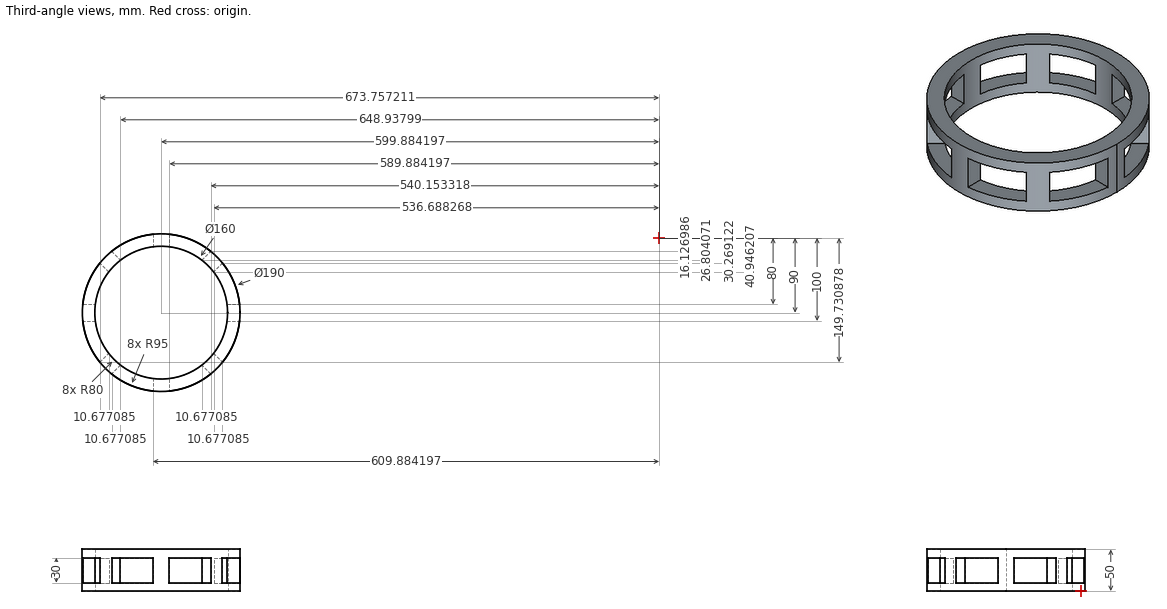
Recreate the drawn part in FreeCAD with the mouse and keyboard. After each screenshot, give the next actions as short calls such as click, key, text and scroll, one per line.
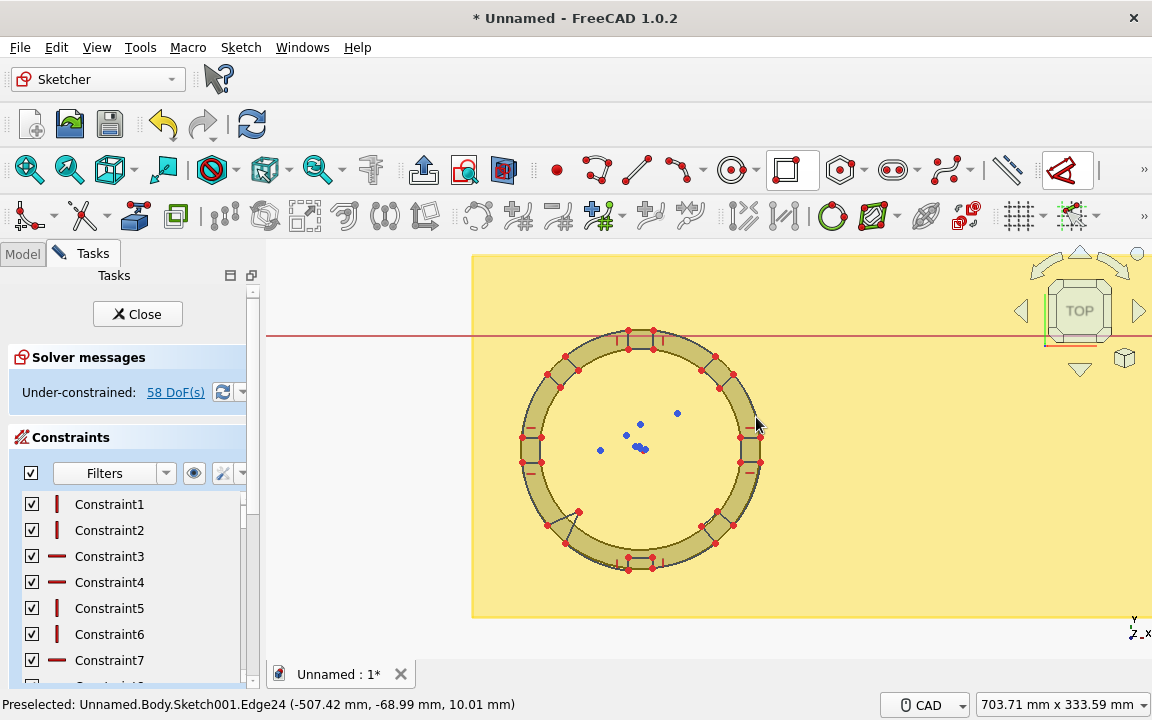
scroll(579, 512, up, 15)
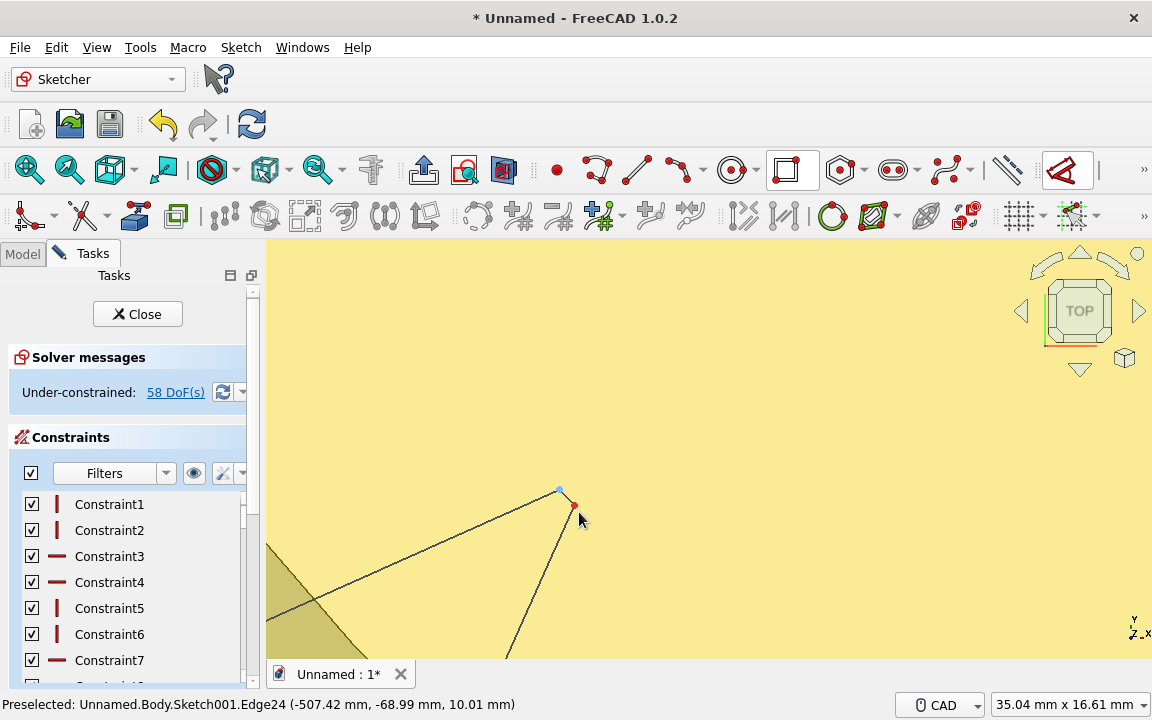
click(567, 497)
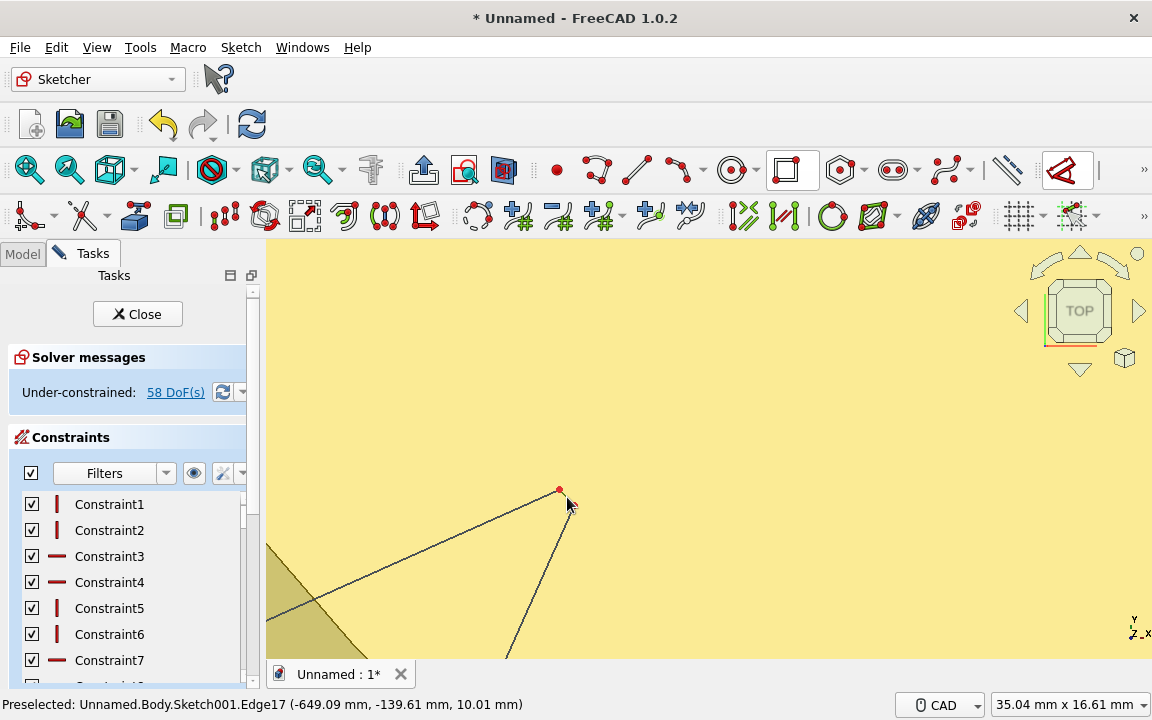
scroll(579, 512, down, 15)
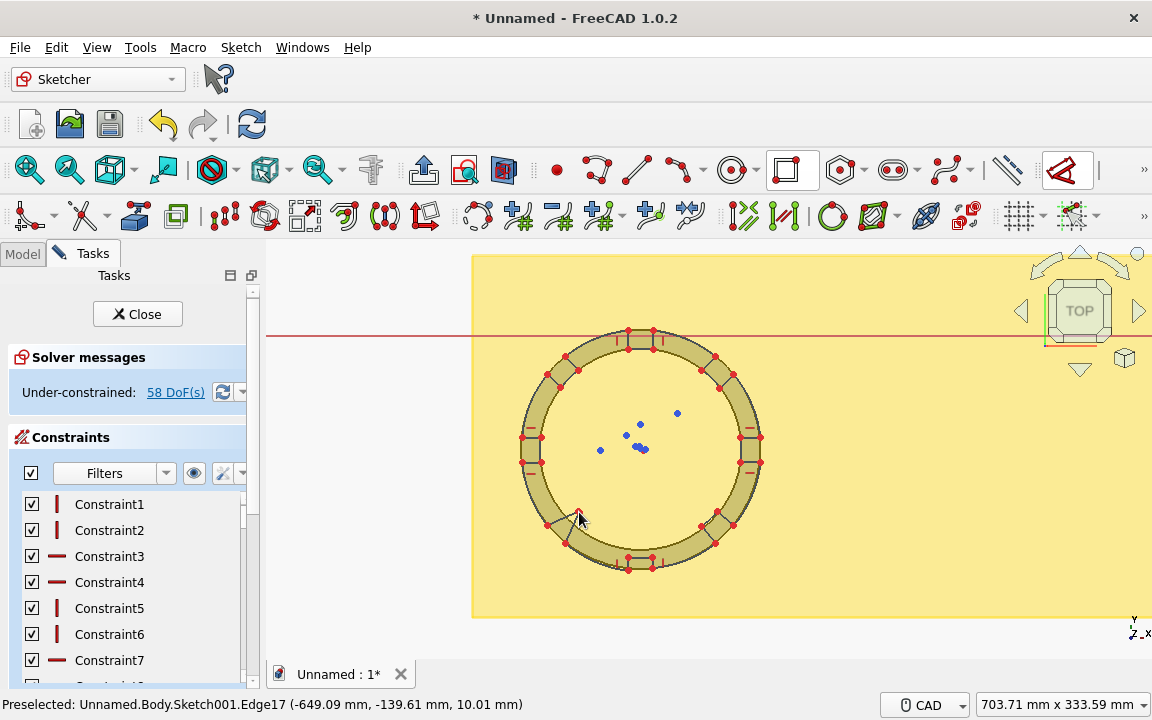
scroll(716, 382, up, 3)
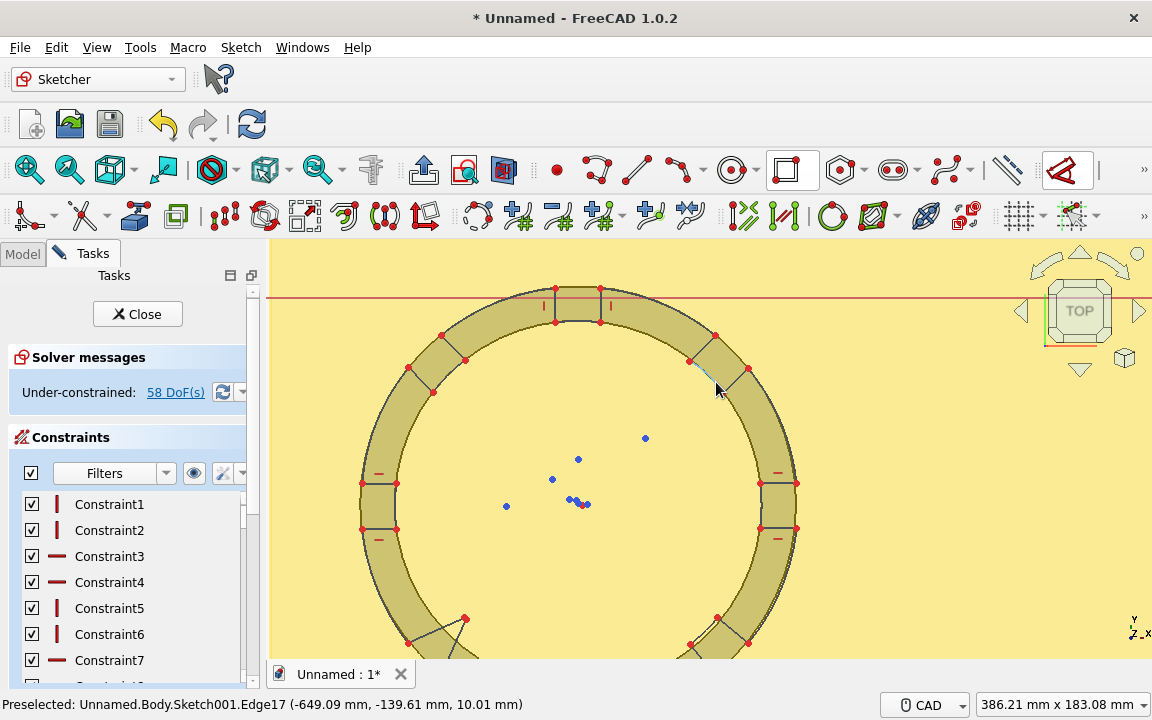
click(715, 382)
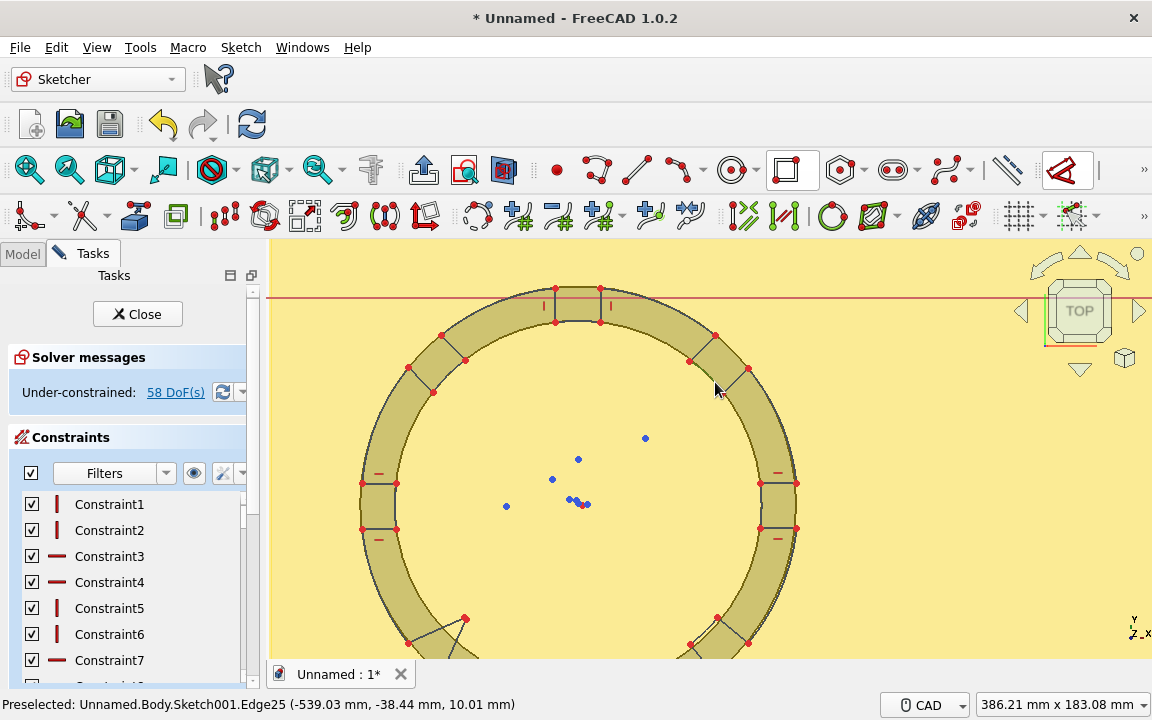
key(c)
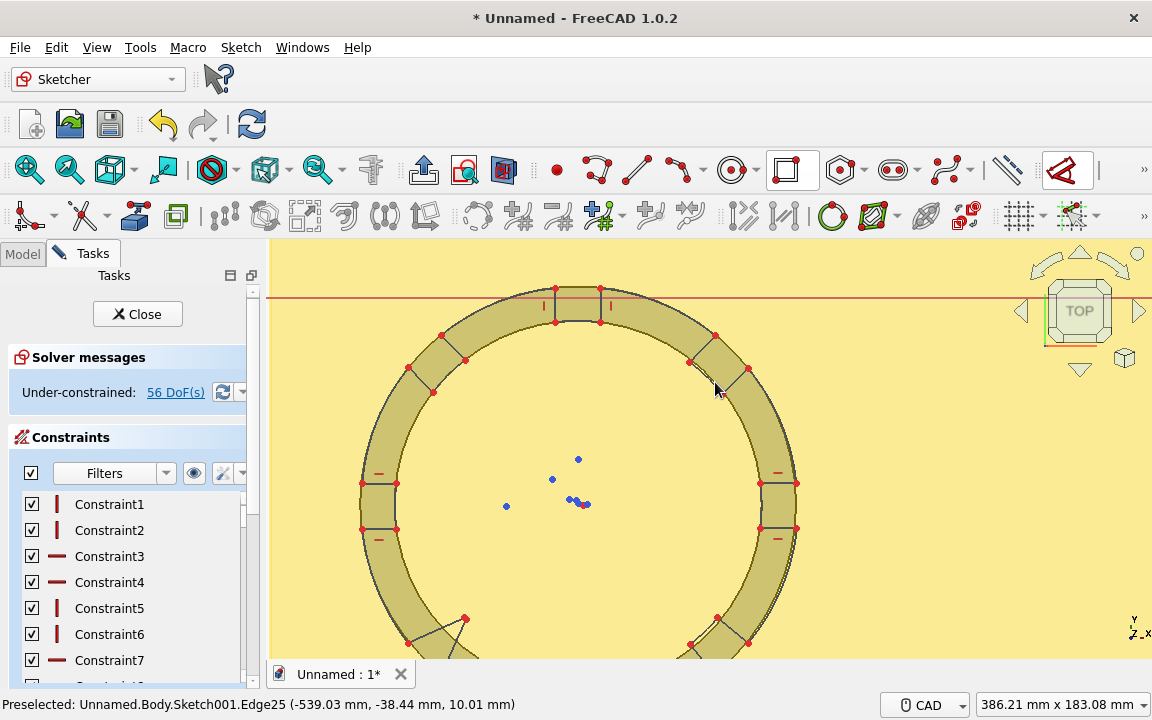
scroll(465, 618, up, 12)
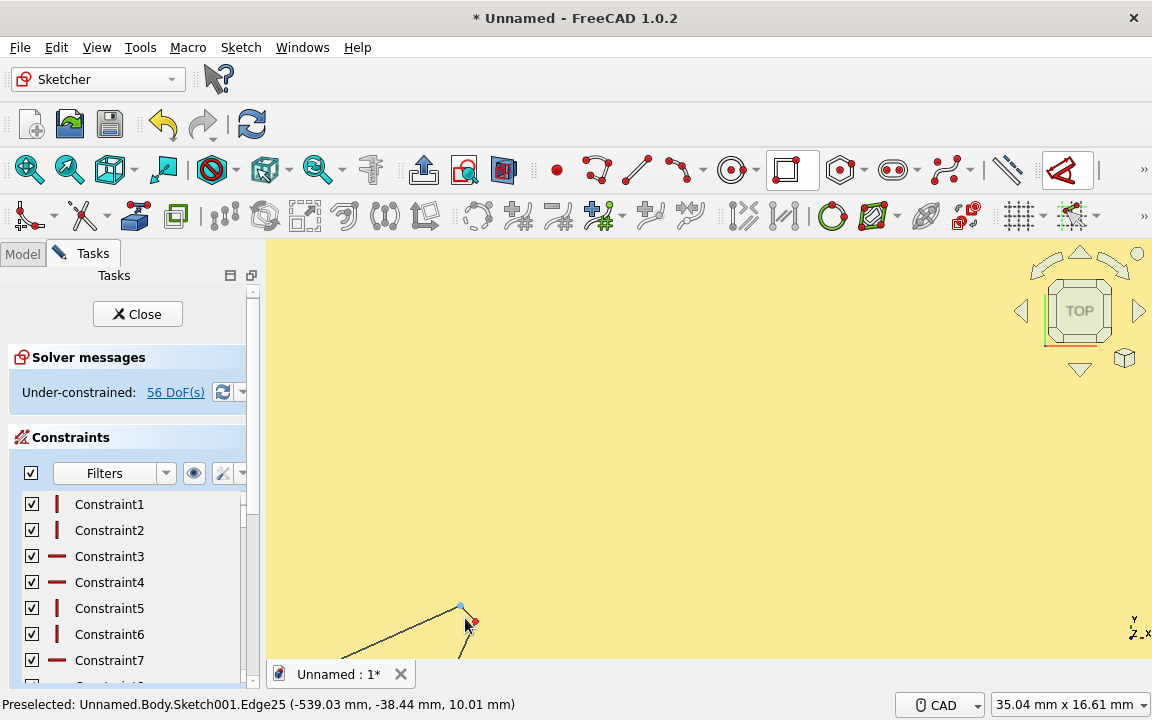
click(468, 613)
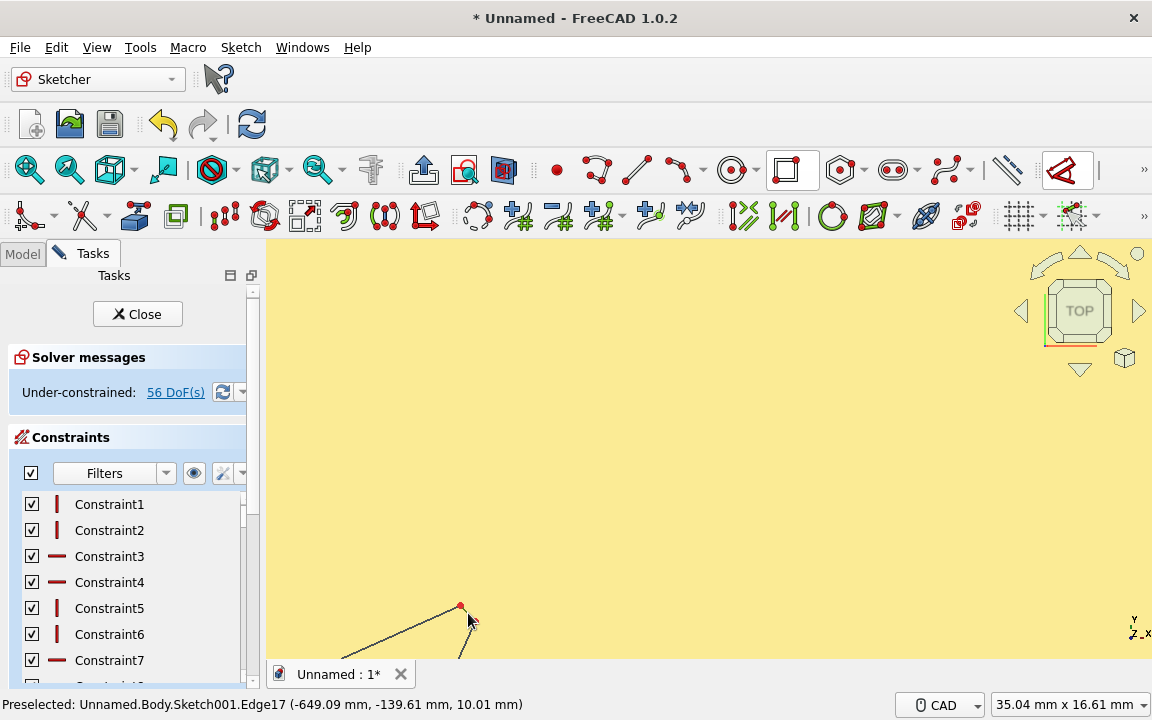
scroll(584, 506, down, 15)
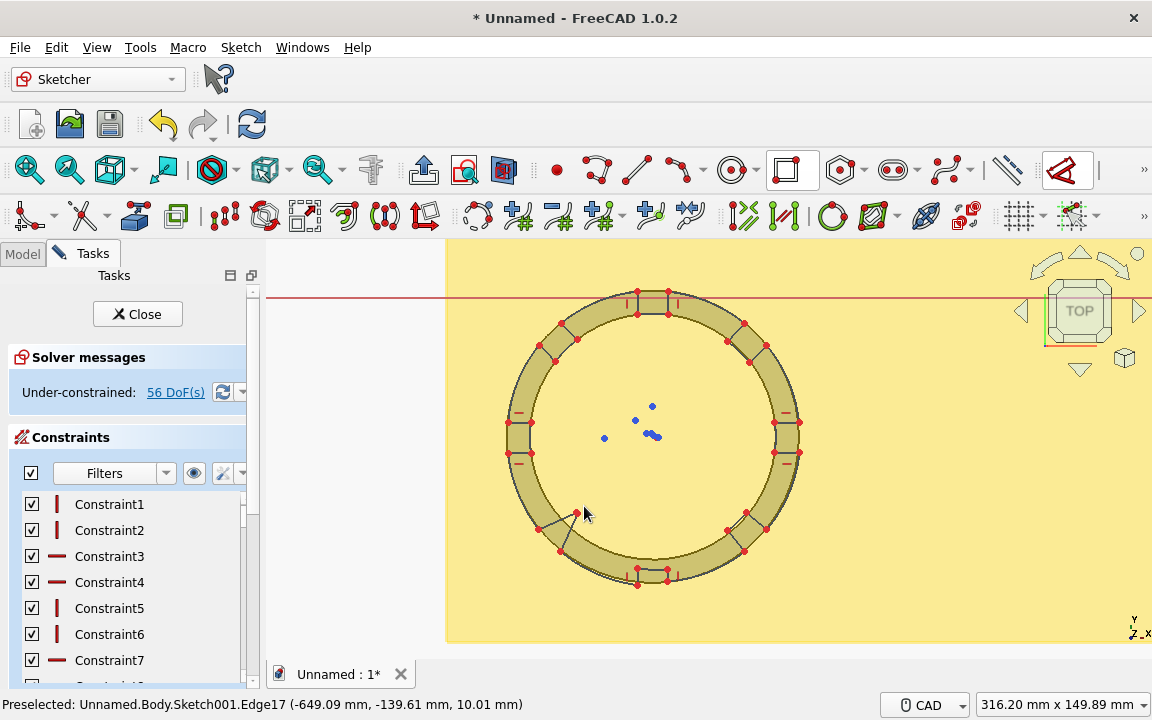
scroll(699, 345, up, 3)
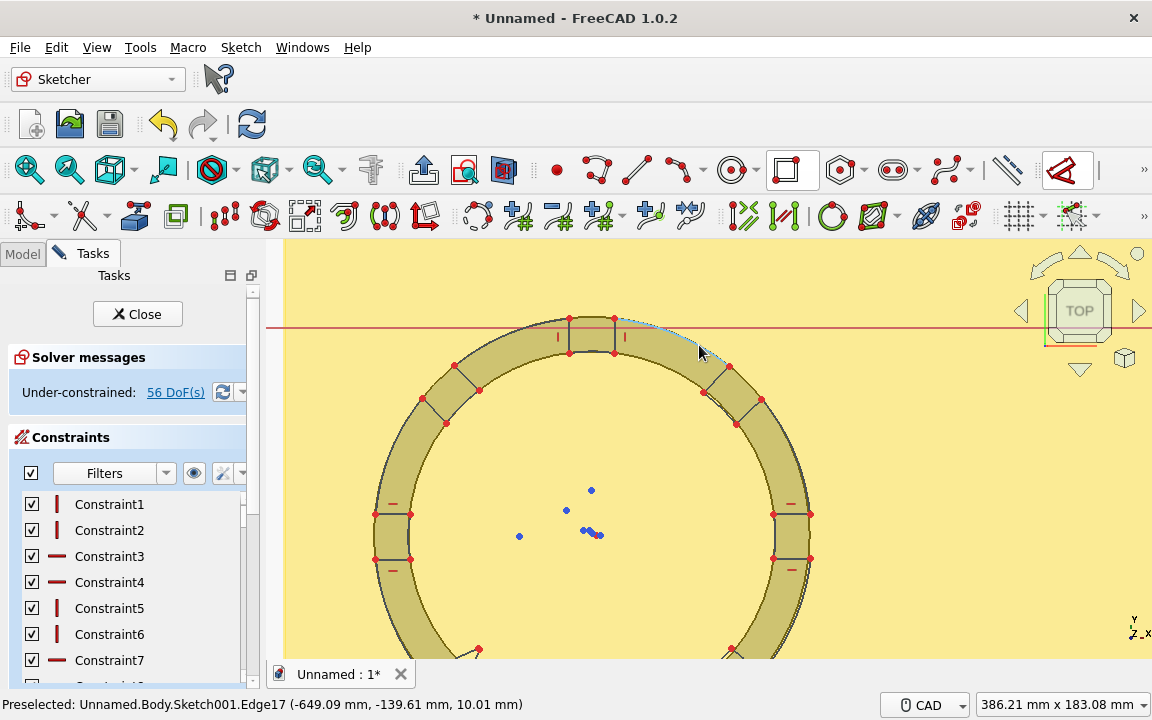
click(698, 345)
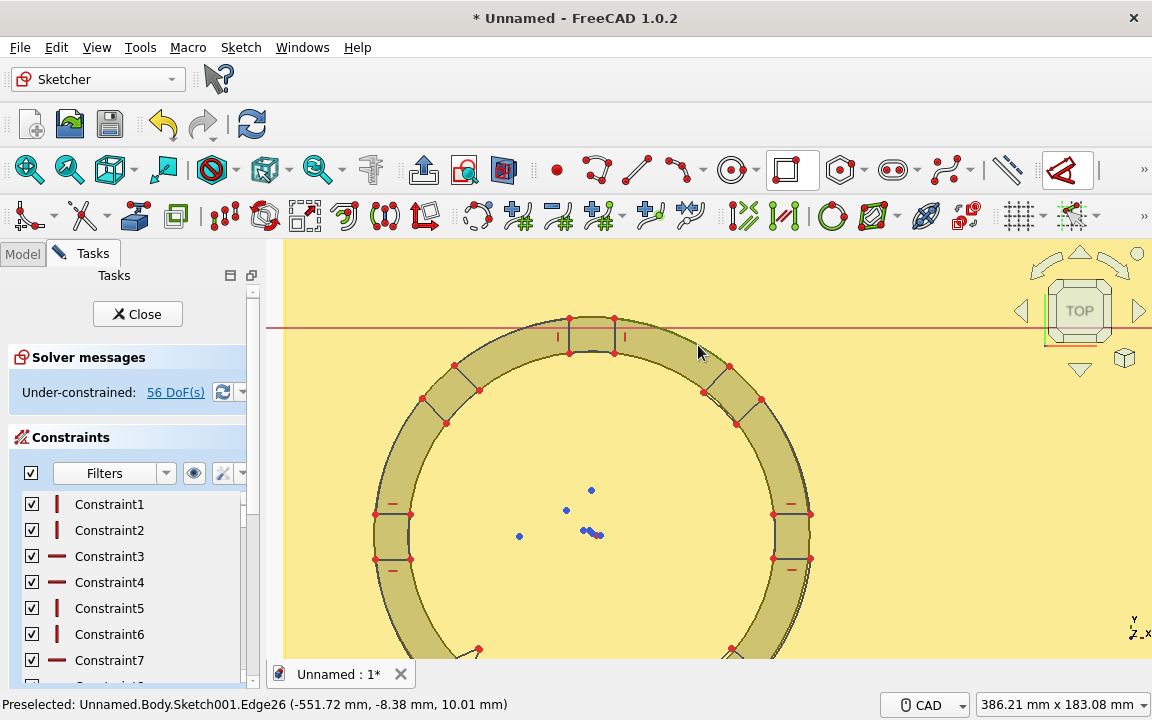
key(c)